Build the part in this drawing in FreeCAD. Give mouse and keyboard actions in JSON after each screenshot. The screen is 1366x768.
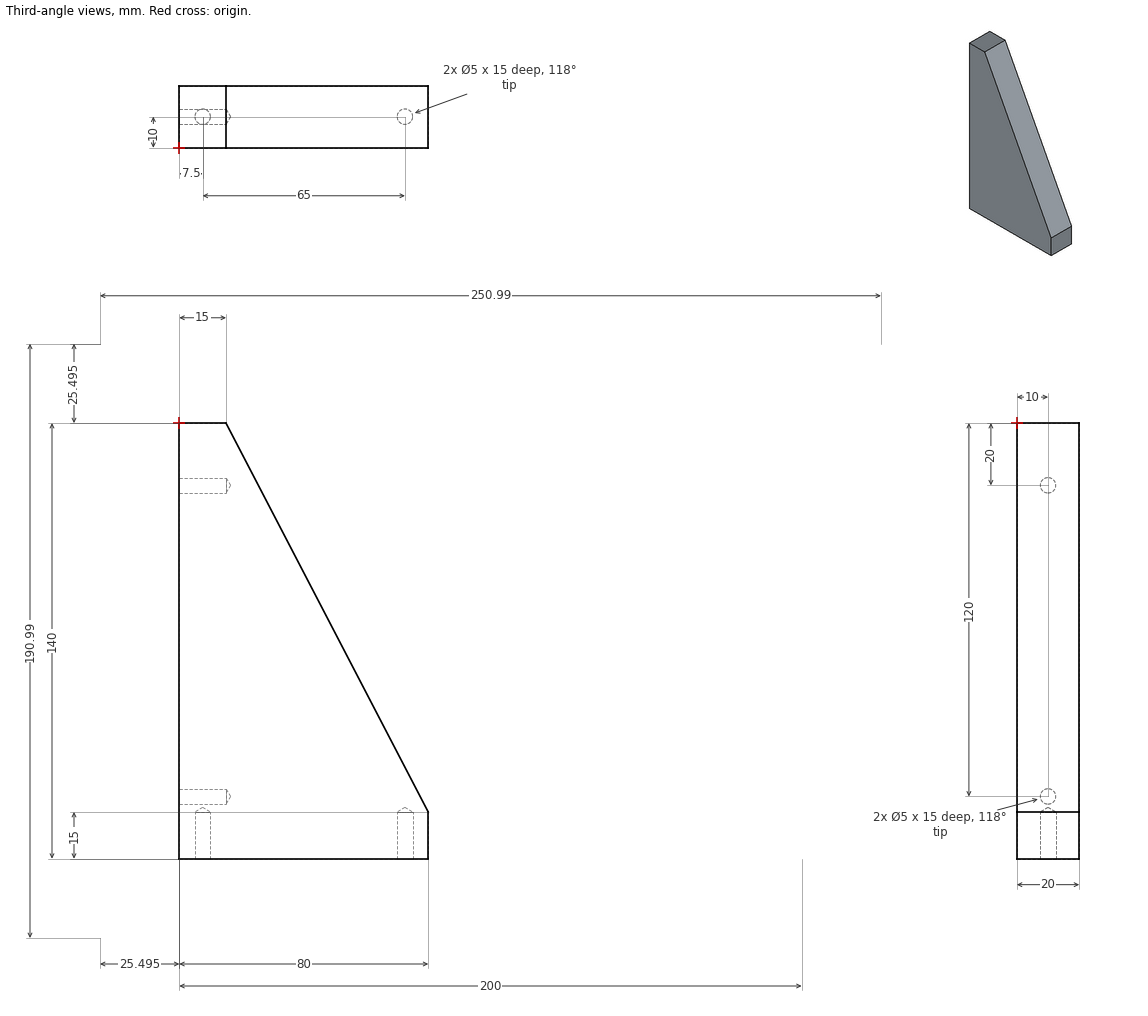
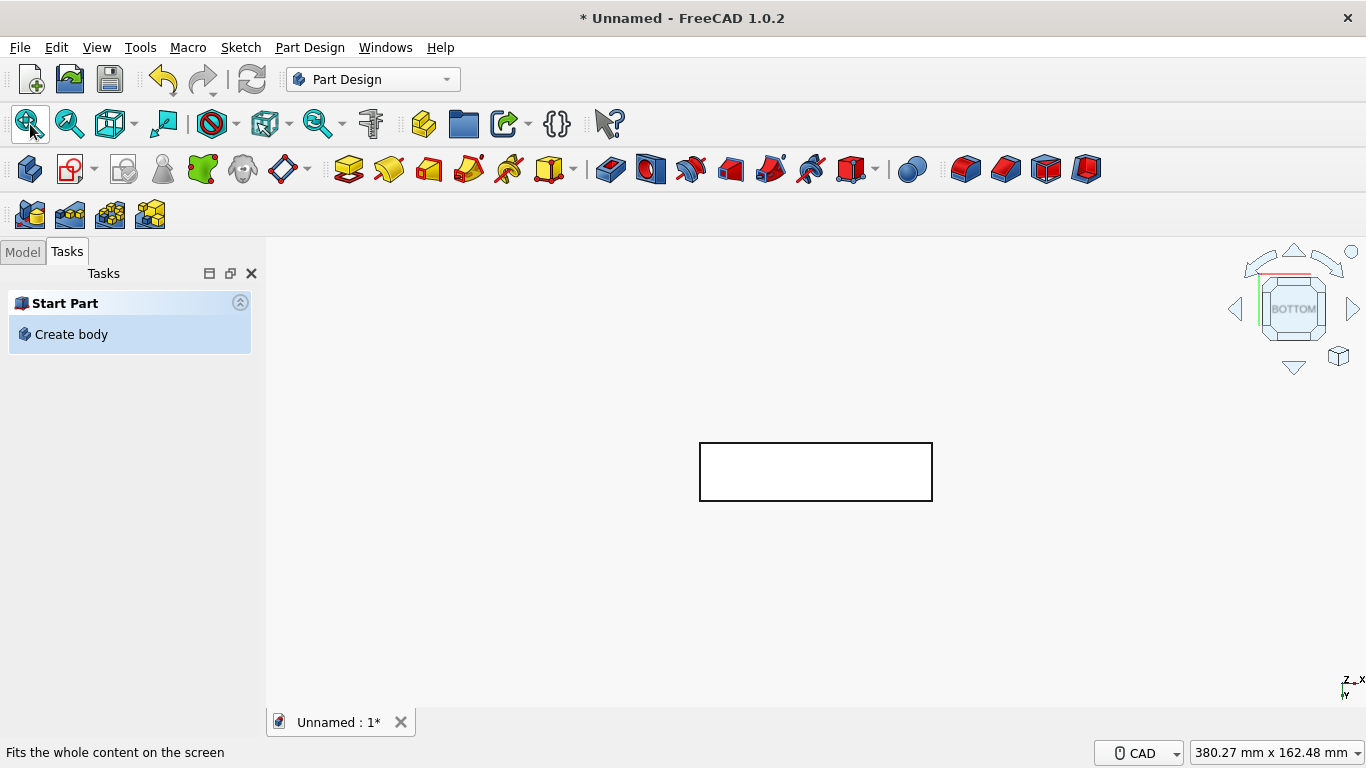
{"action": "left_click", "coordinate": [882, 471]}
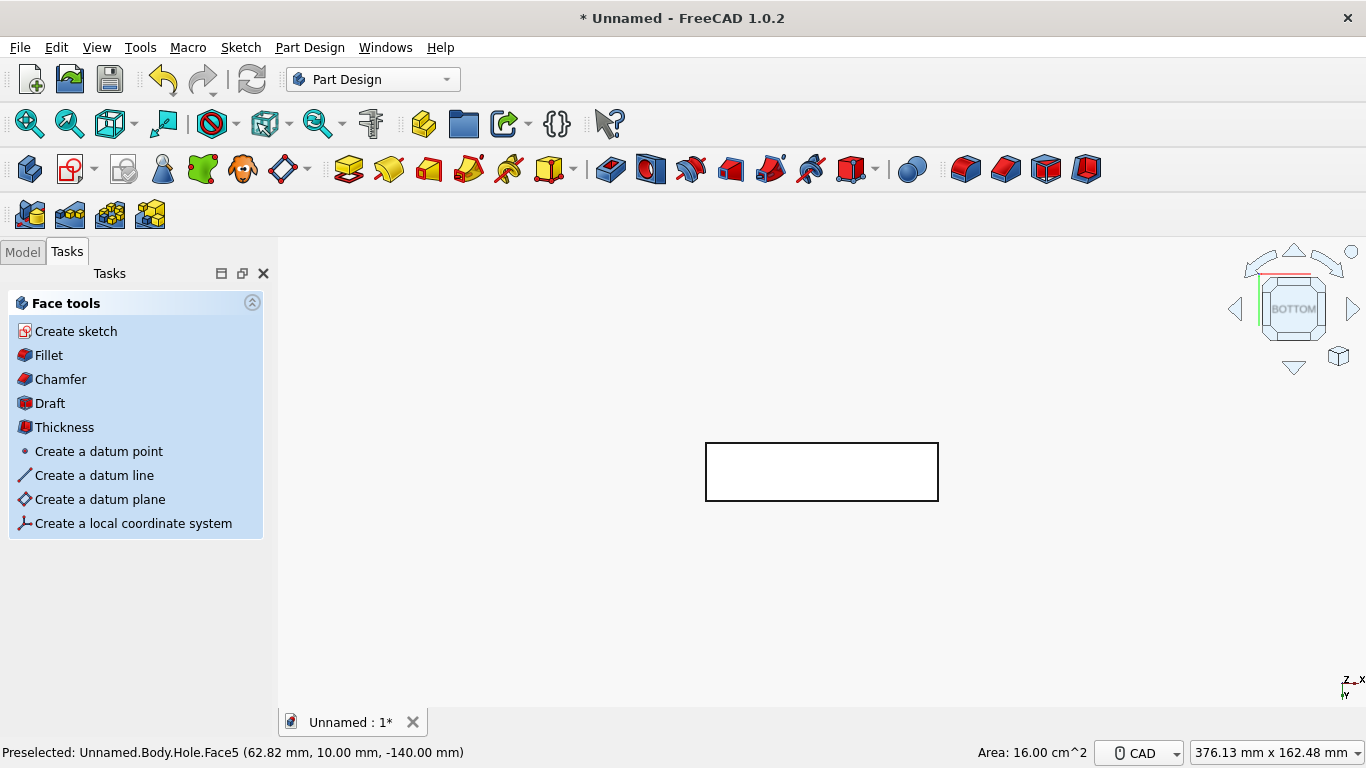
{"action": "left_click", "coordinate": [70, 170]}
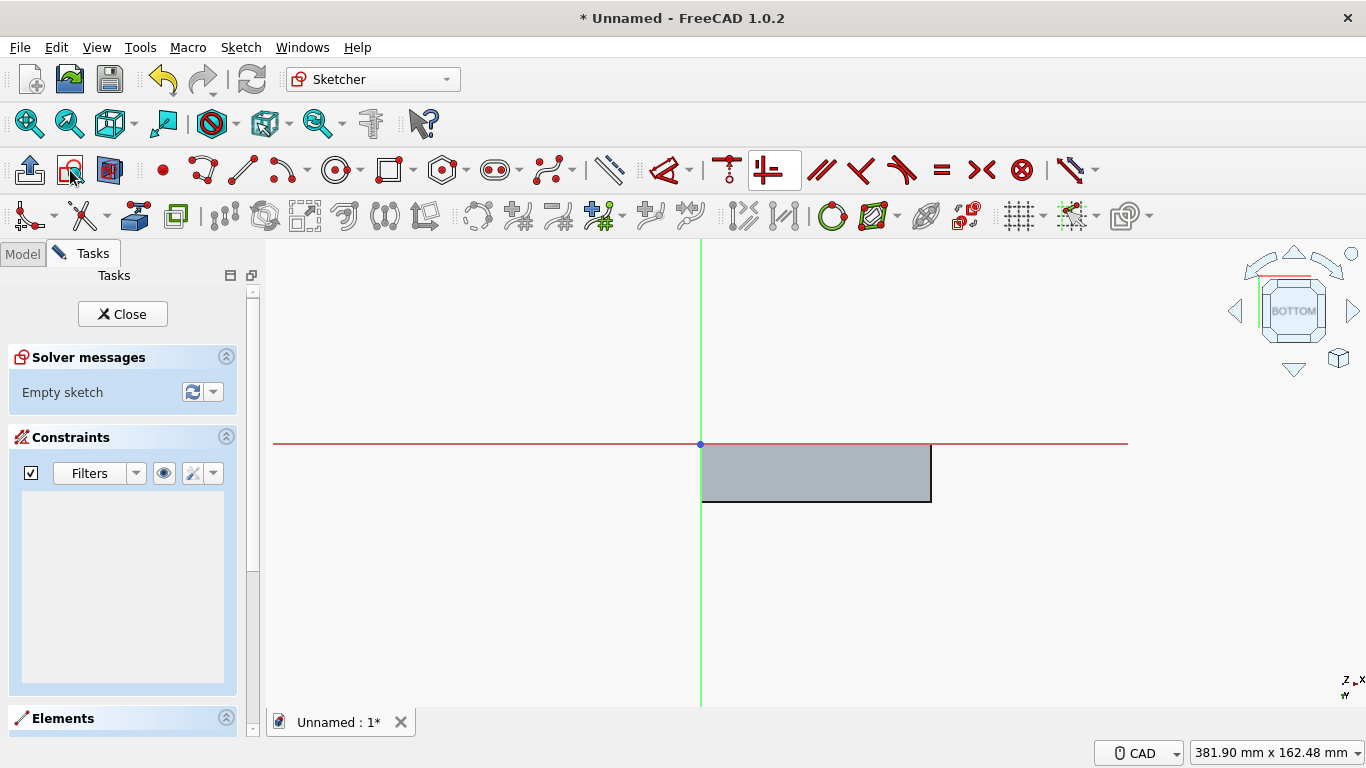
{"action": "scroll", "coordinate": [844, 456], "scroll_direction": "up", "scroll_amount": 5}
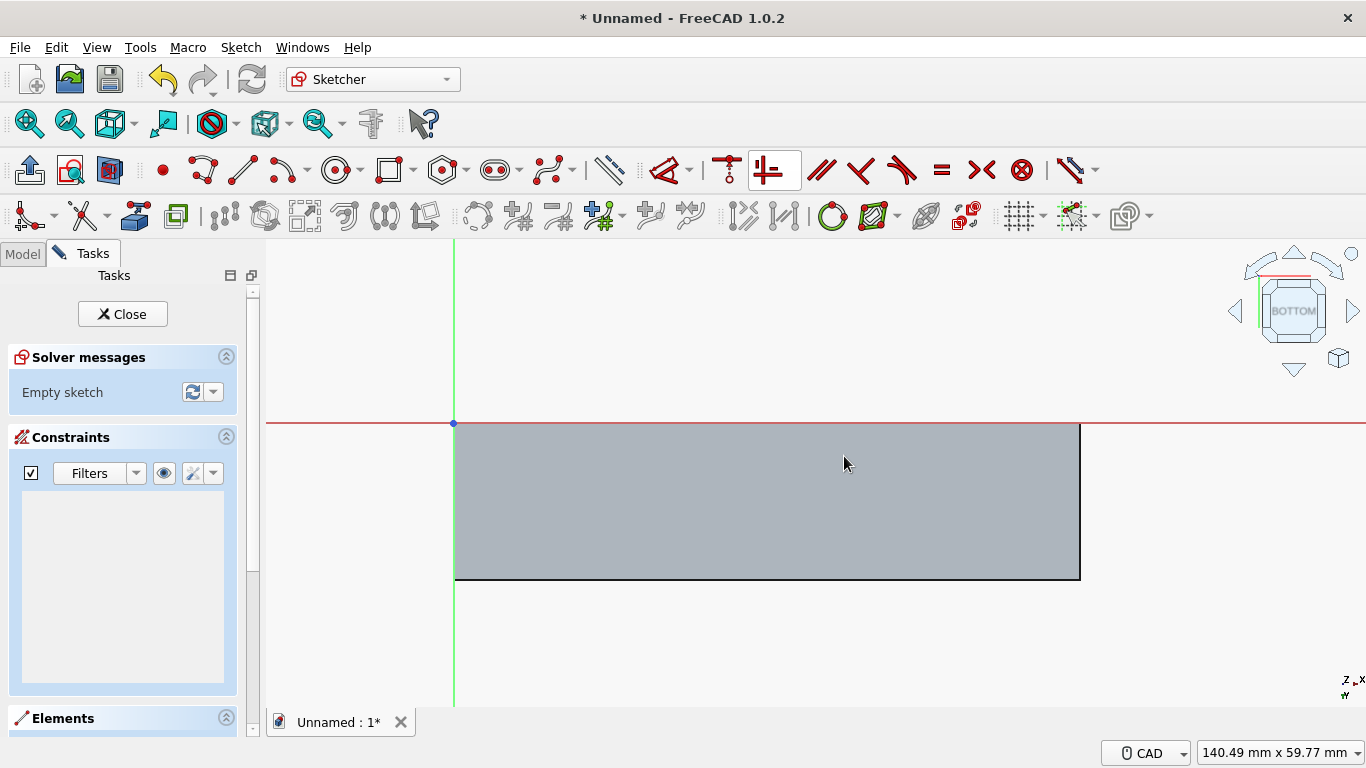
{"action": "left_click", "coordinate": [336, 170]}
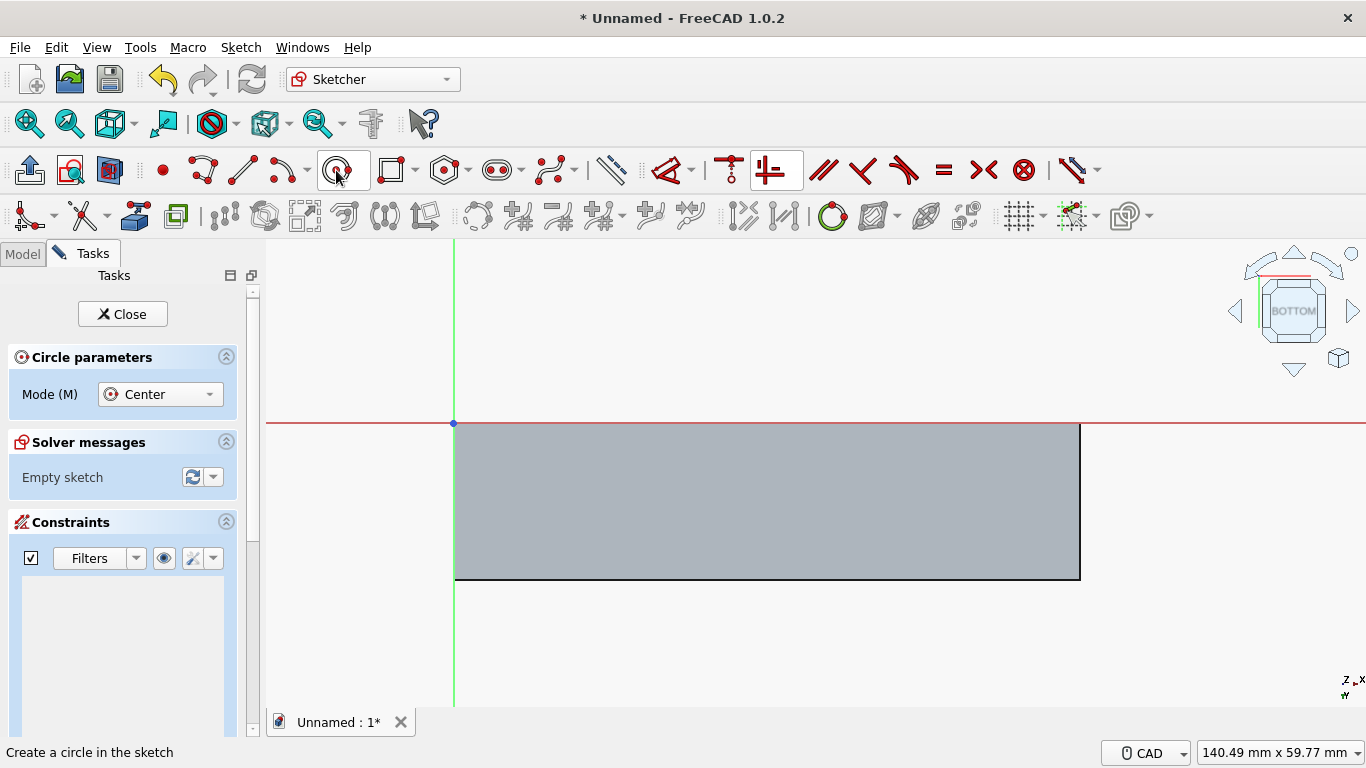
{"action": "left_click", "coordinate": [1021, 501]}
{"action": "left_click", "coordinate": [1035, 488]}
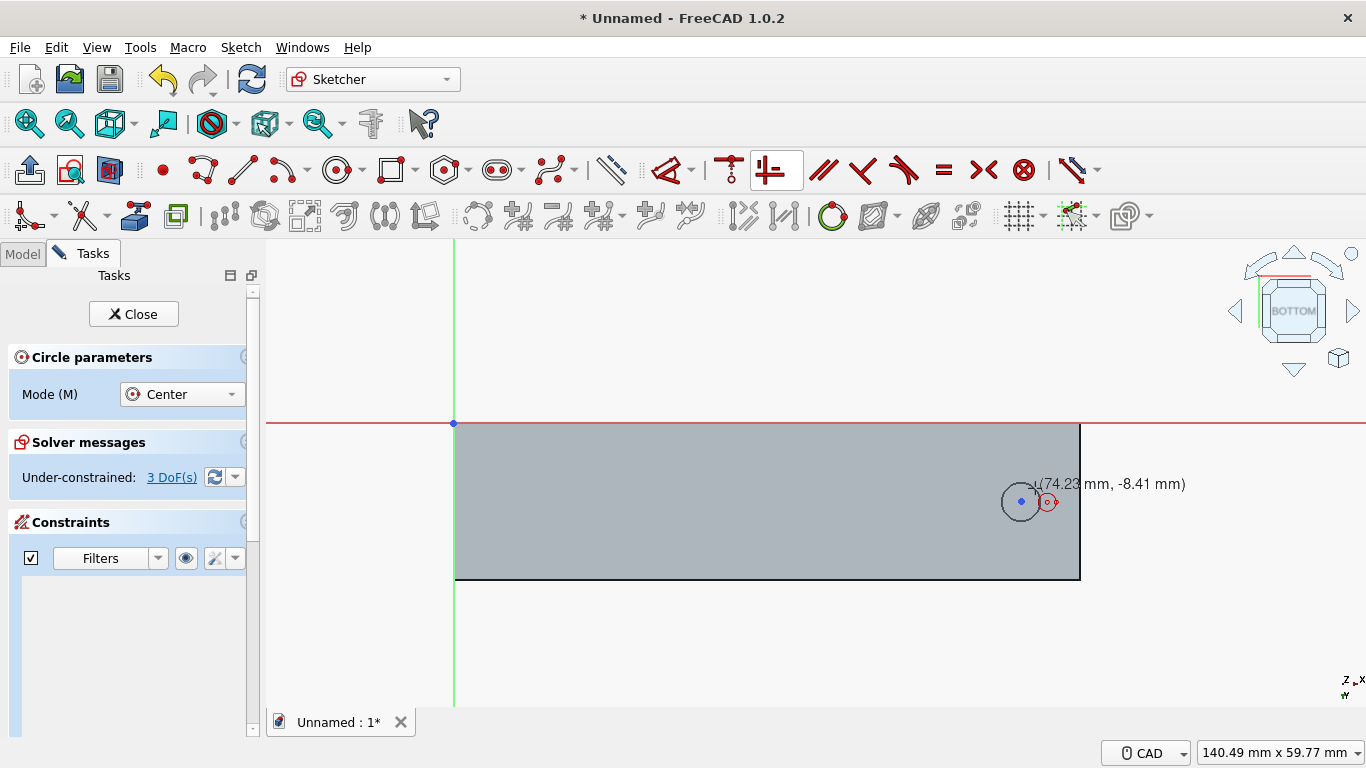
{"action": "left_click", "coordinate": [513, 501]}
{"action": "left_click", "coordinate": [526, 488]}
{"action": "key", "text": "Escape"}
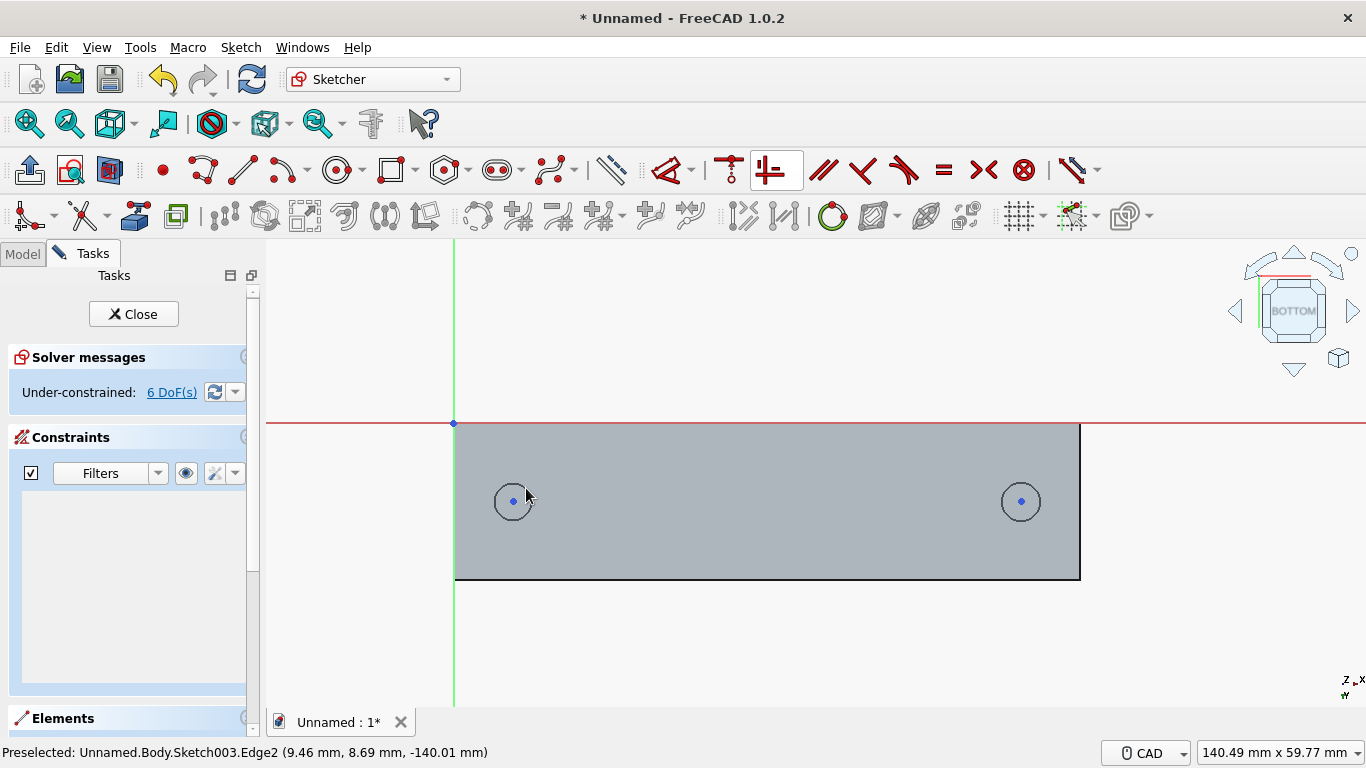
{"action": "left_click", "coordinate": [1034, 488]}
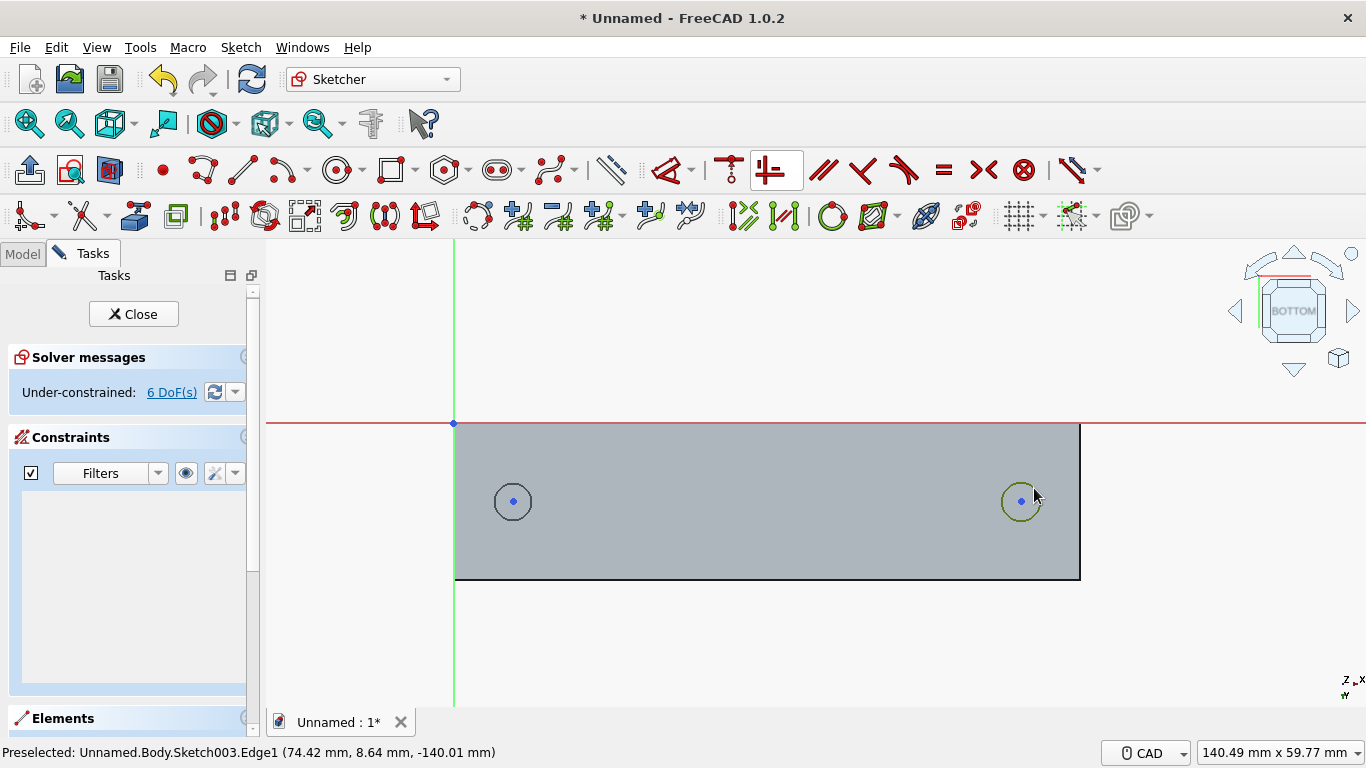
{"action": "left_click", "coordinate": [526, 489]}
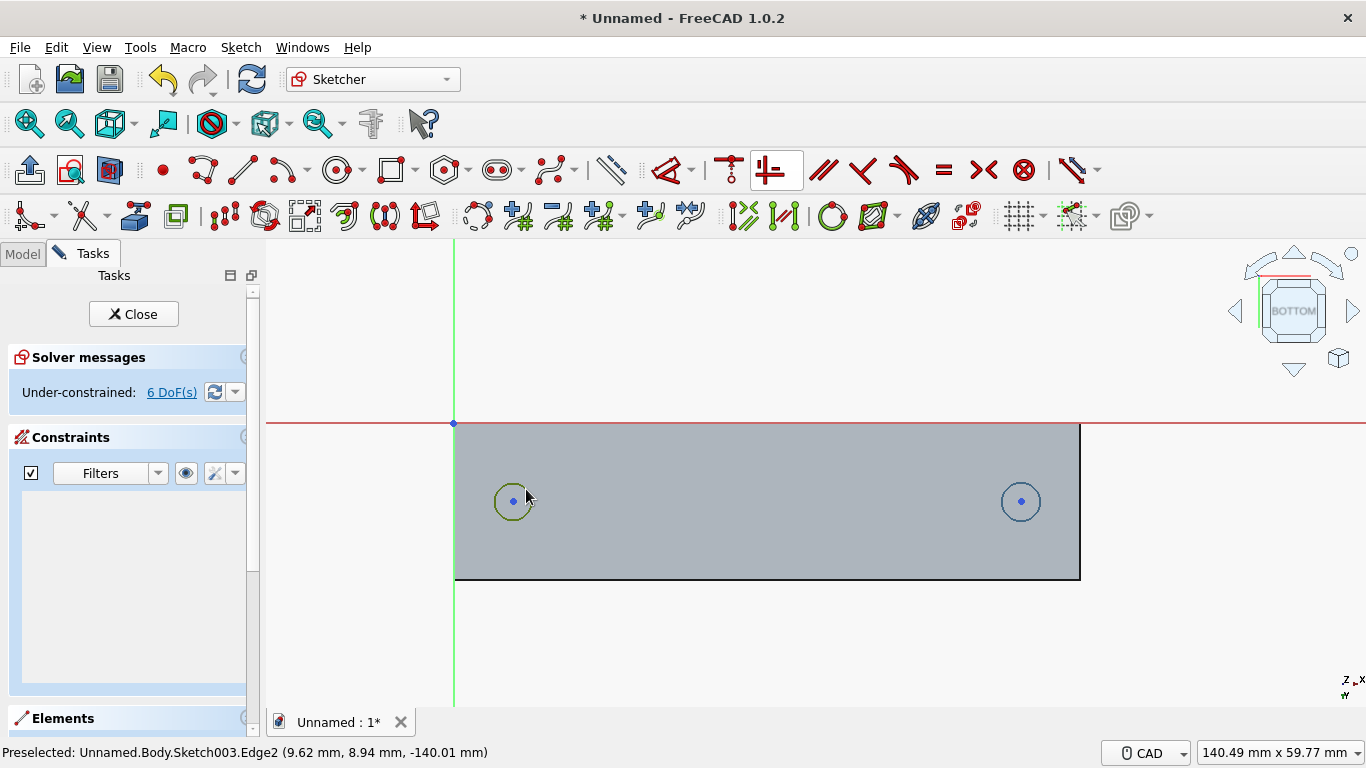
{"action": "left_click", "coordinate": [944, 170]}